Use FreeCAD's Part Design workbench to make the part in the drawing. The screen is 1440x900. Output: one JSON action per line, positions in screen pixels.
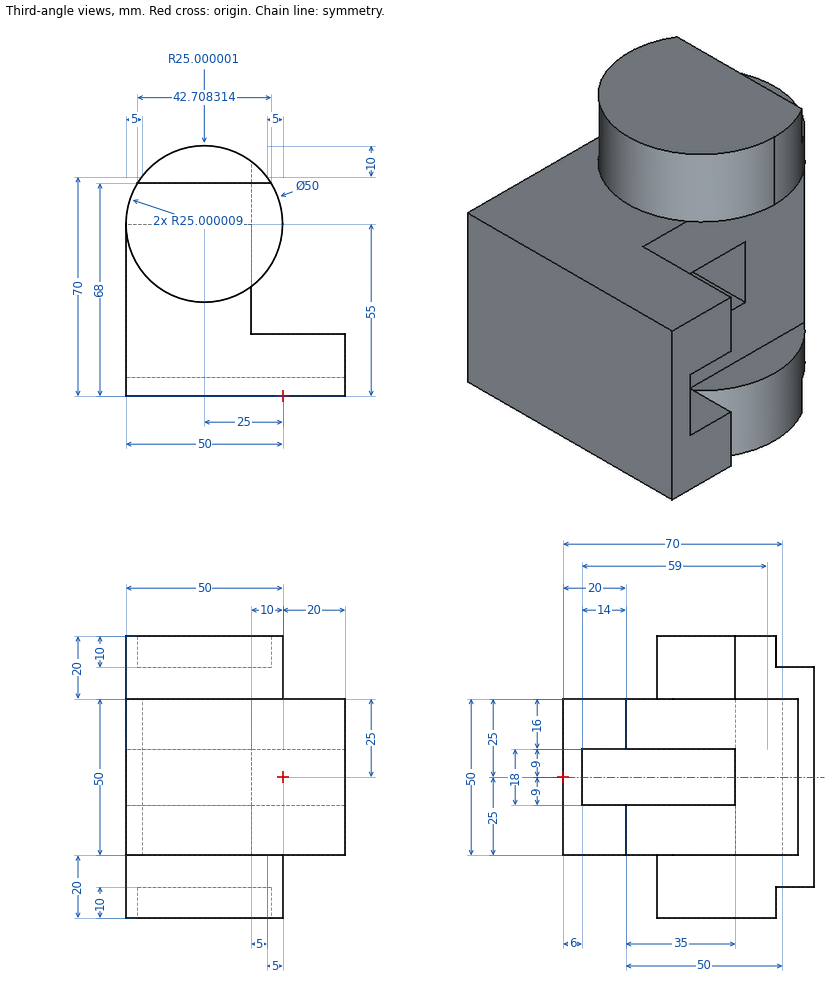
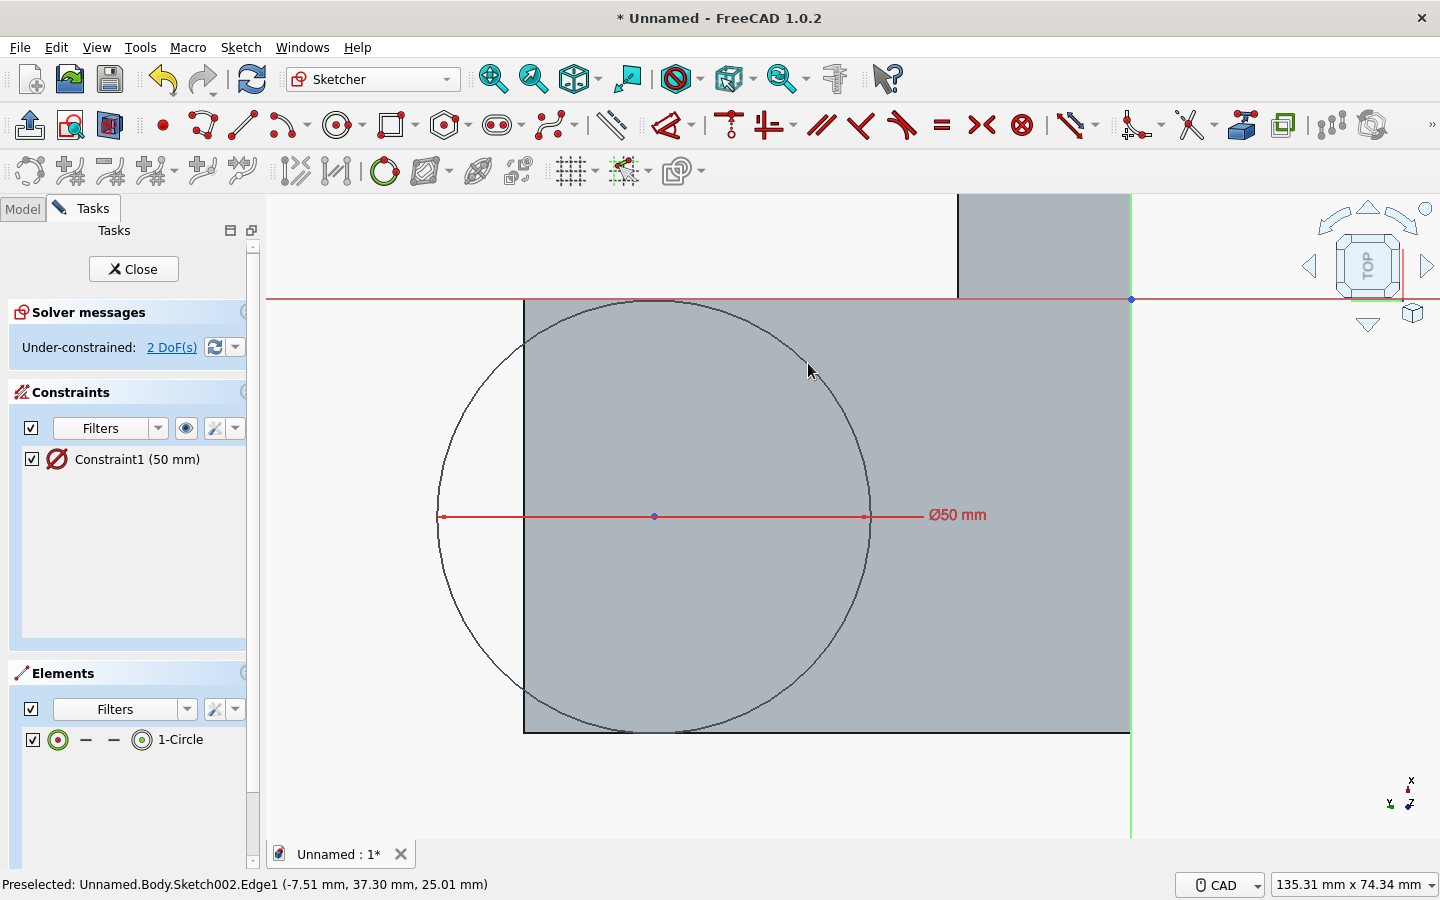
{"action": "left_click", "coordinate": [666, 126]}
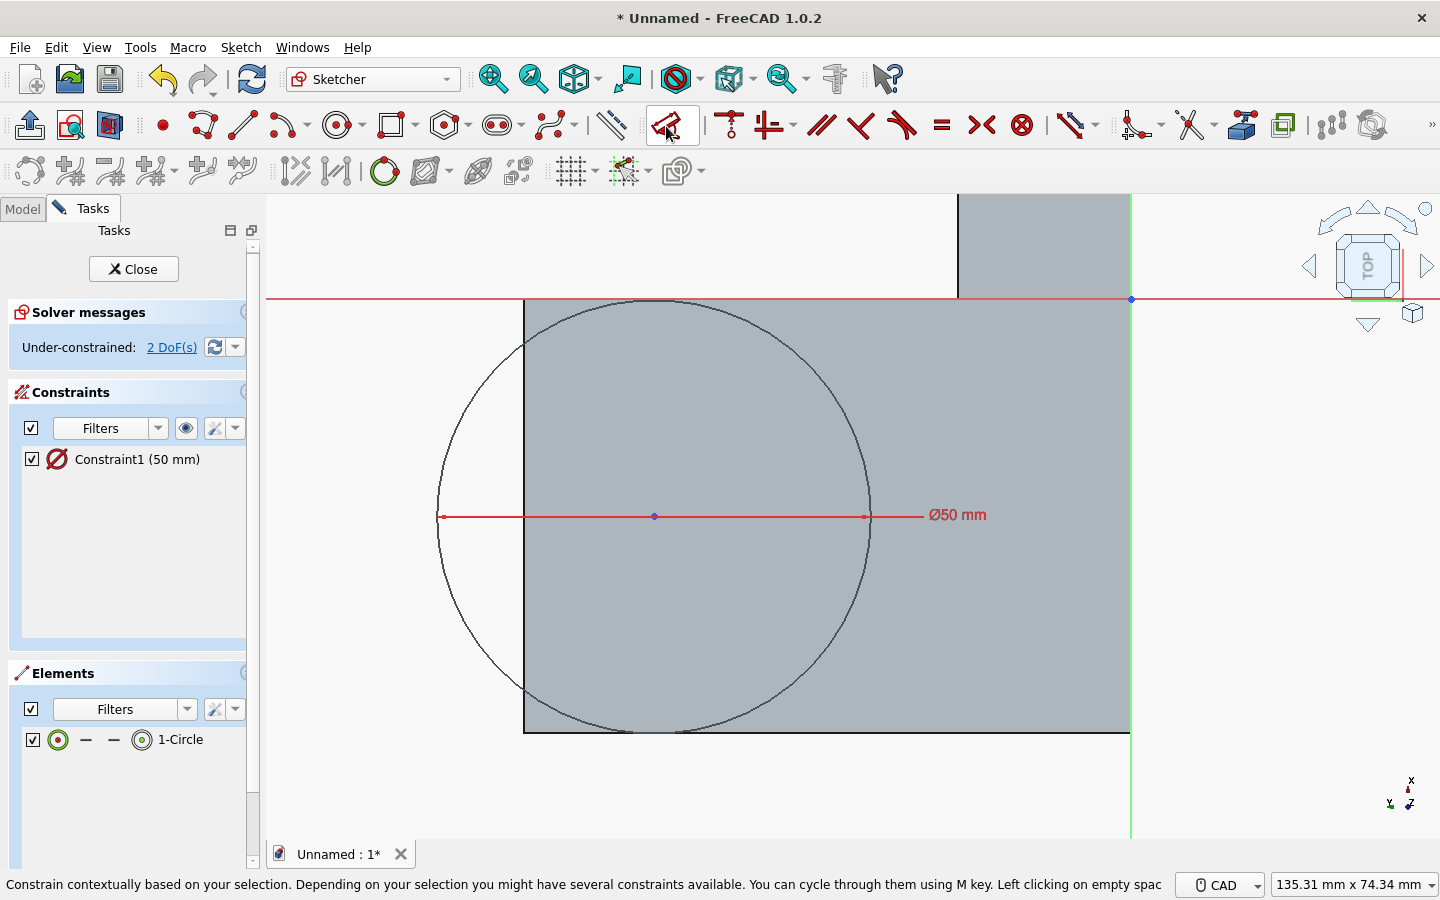
{"action": "left_click", "coordinate": [654, 517]}
{"action": "left_click", "coordinate": [893, 265]}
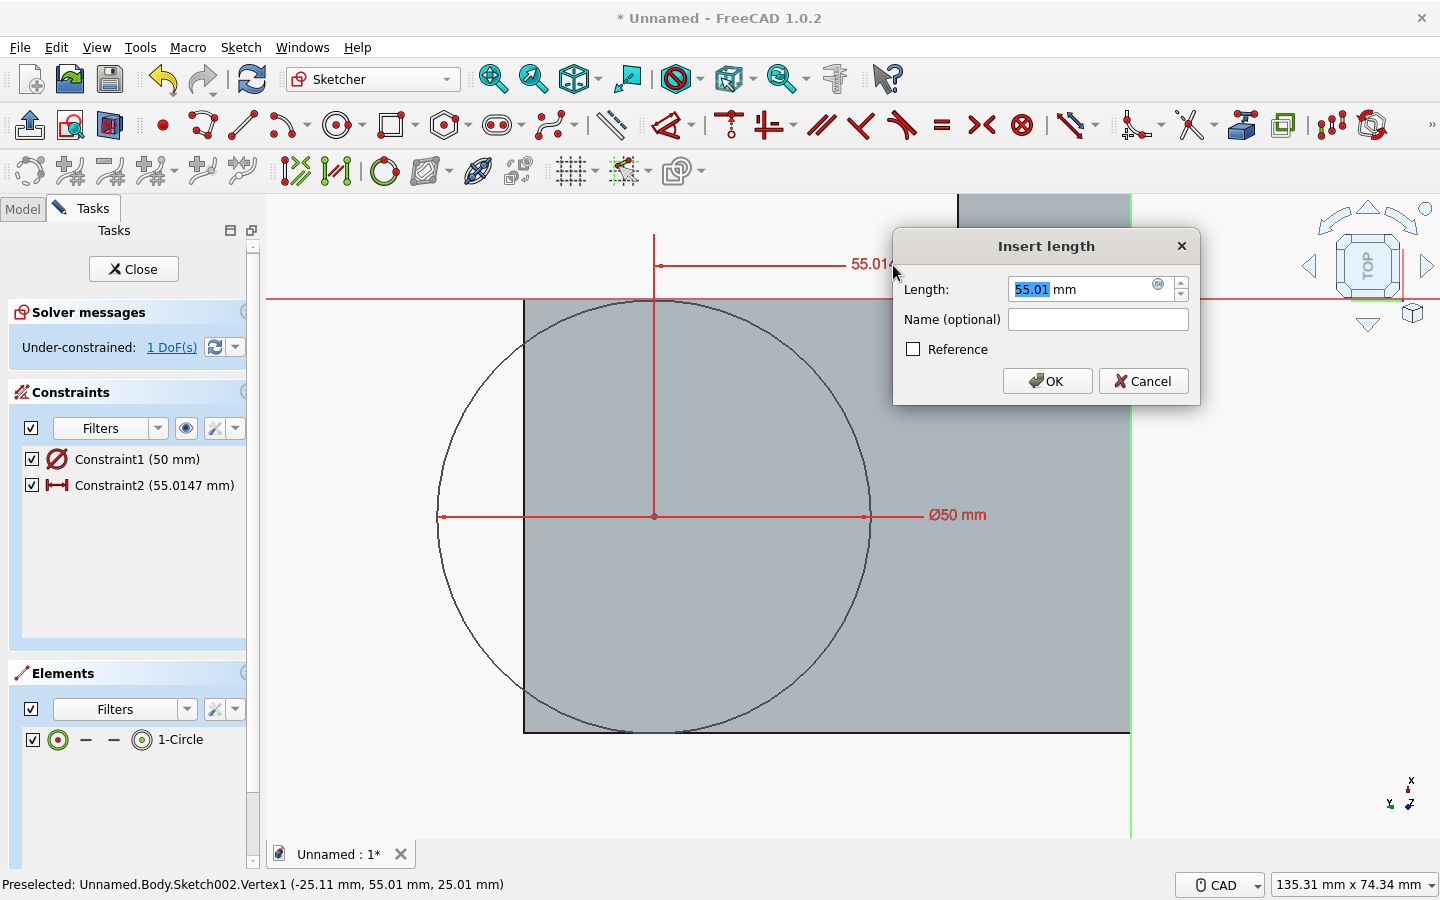
{"action": "type", "text": "55"}
{"action": "key", "text": "Return"}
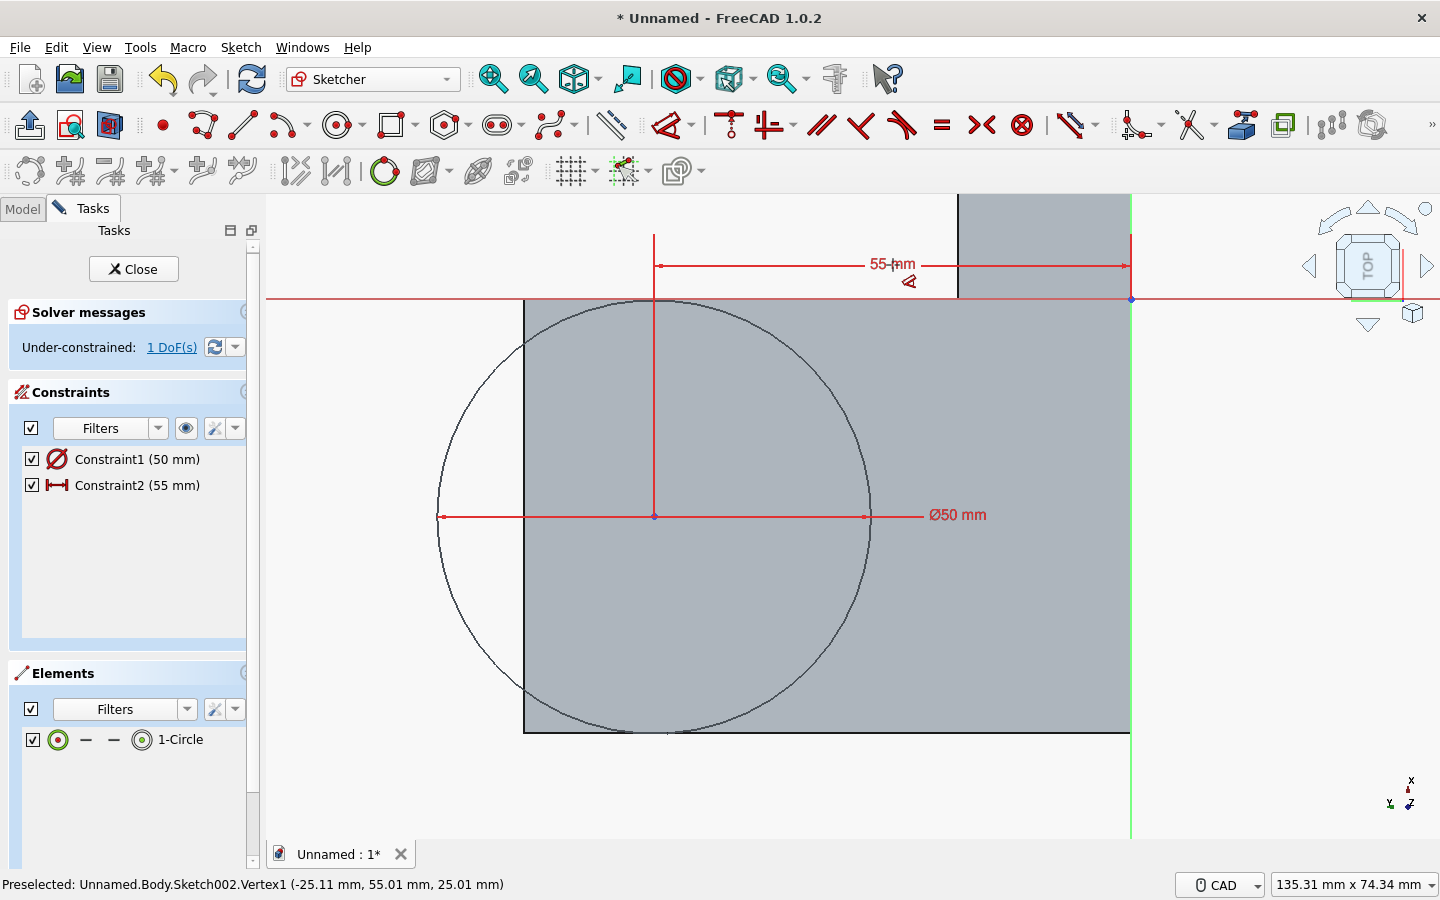
{"action": "left_click", "coordinate": [654, 517]}
{"action": "left_click", "coordinate": [1165, 408]}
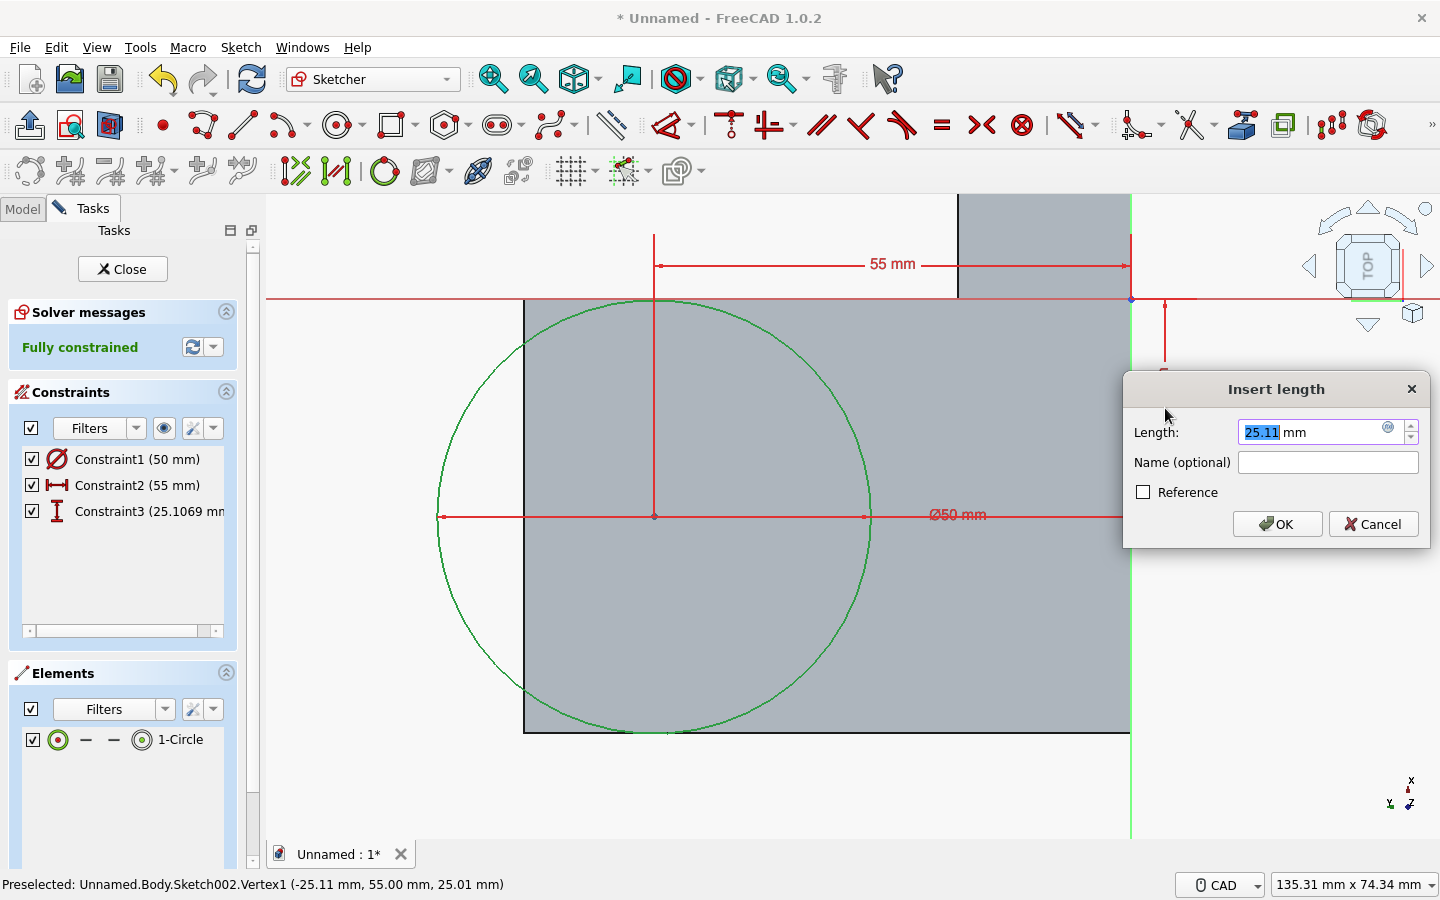
{"action": "type", "text": "25"}
{"action": "key", "text": "Return"}
{"action": "key", "text": "Escape"}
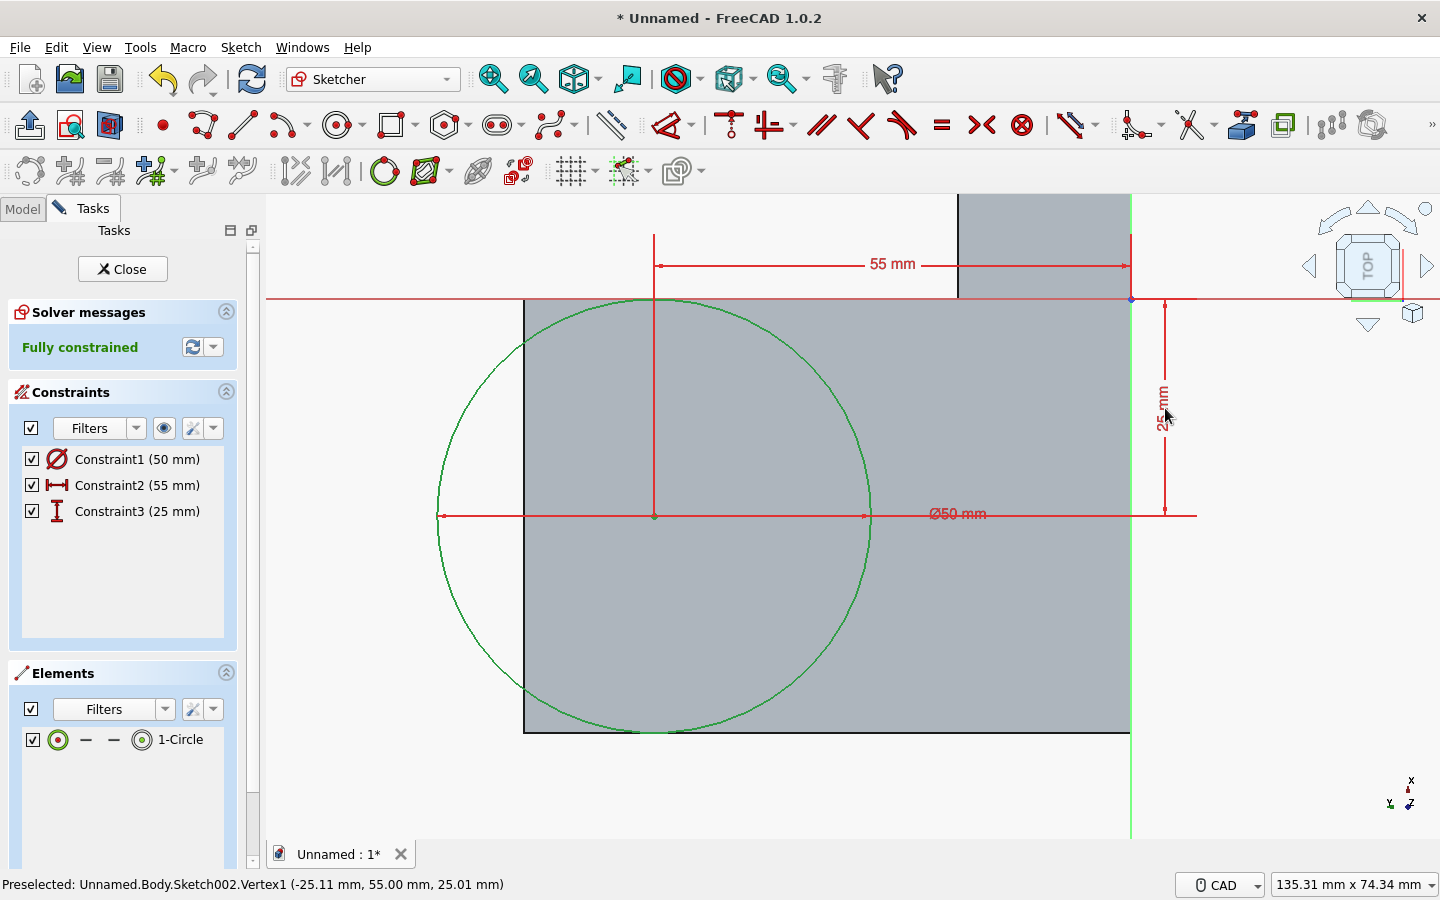
{"action": "left_click", "coordinate": [123, 269]}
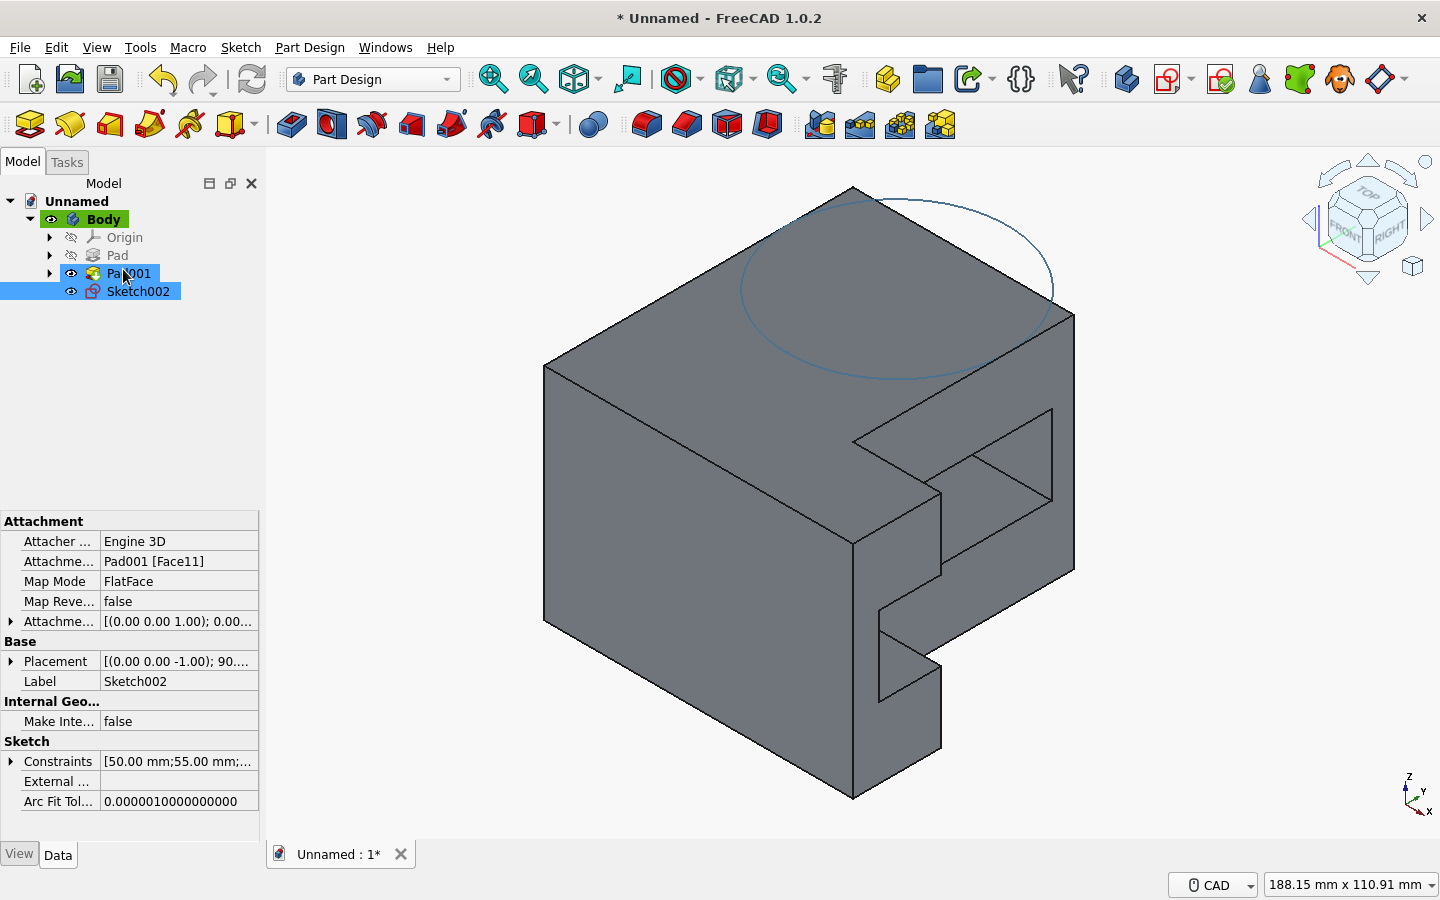
{"action": "left_click", "coordinate": [30, 124]}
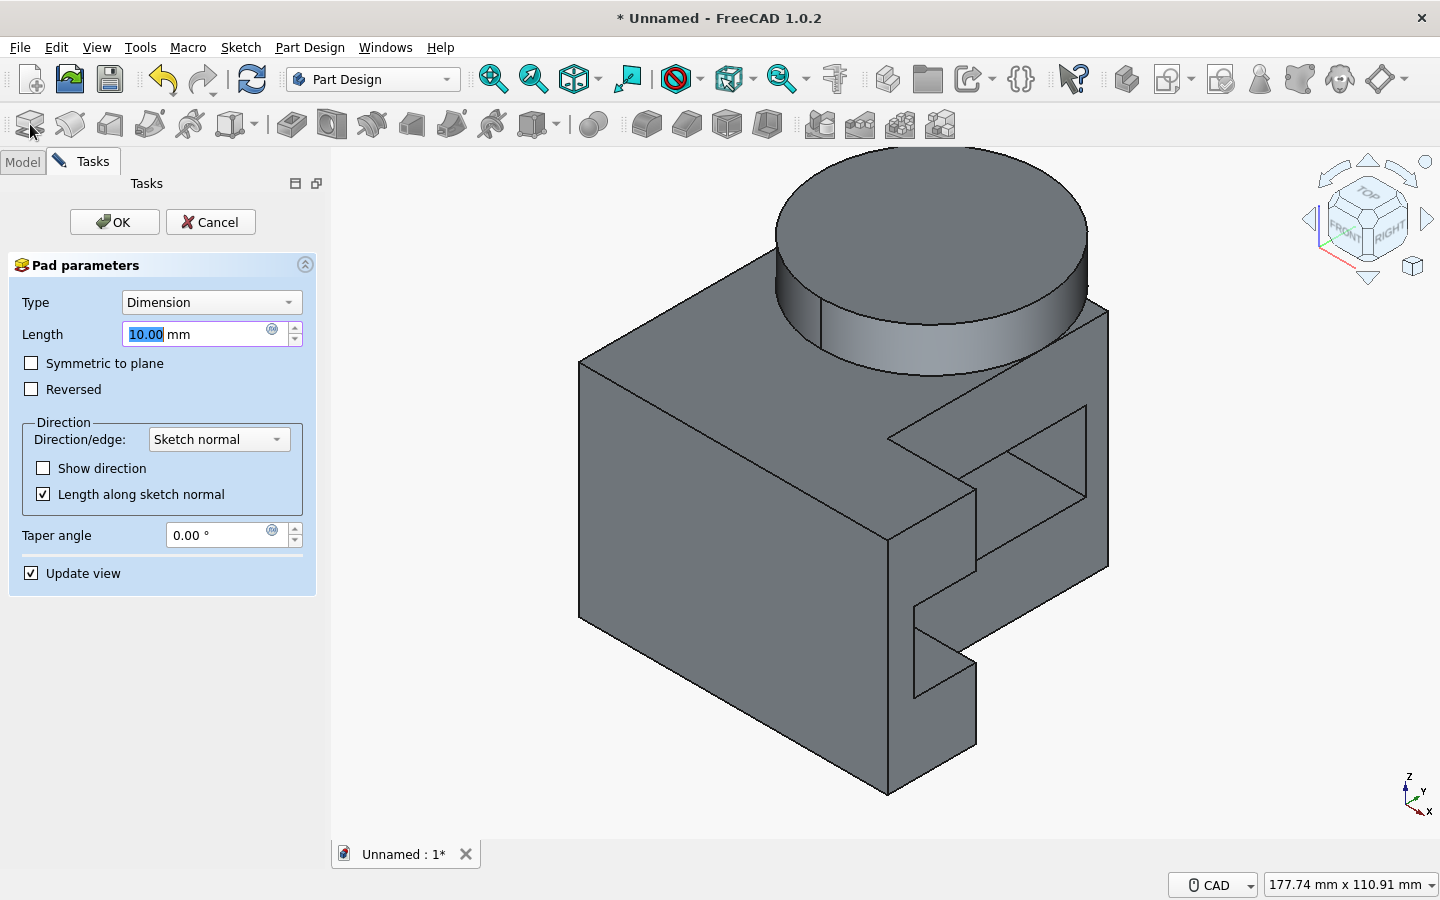
{"action": "type", "text": "50"}
{"action": "key", "text": "Tab"}